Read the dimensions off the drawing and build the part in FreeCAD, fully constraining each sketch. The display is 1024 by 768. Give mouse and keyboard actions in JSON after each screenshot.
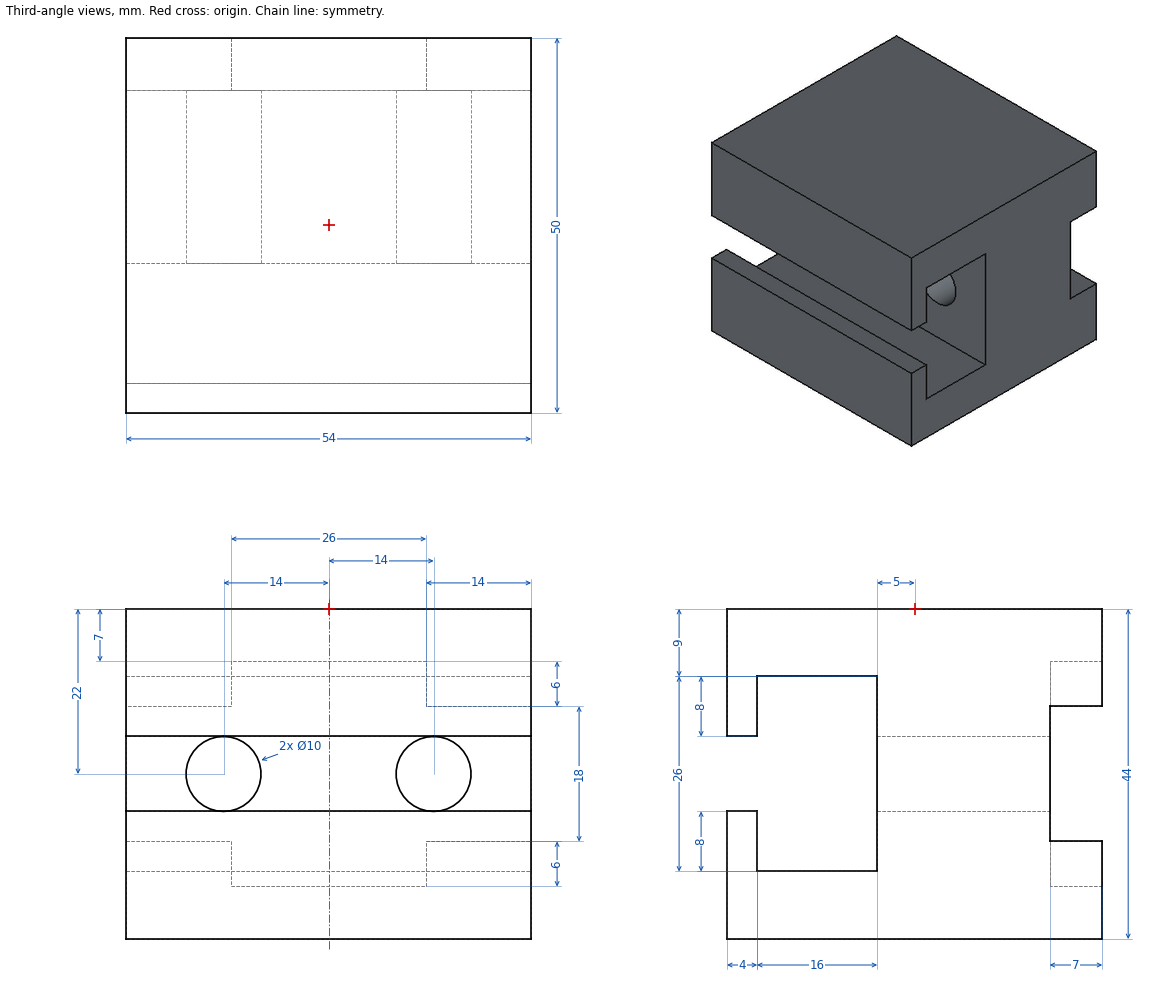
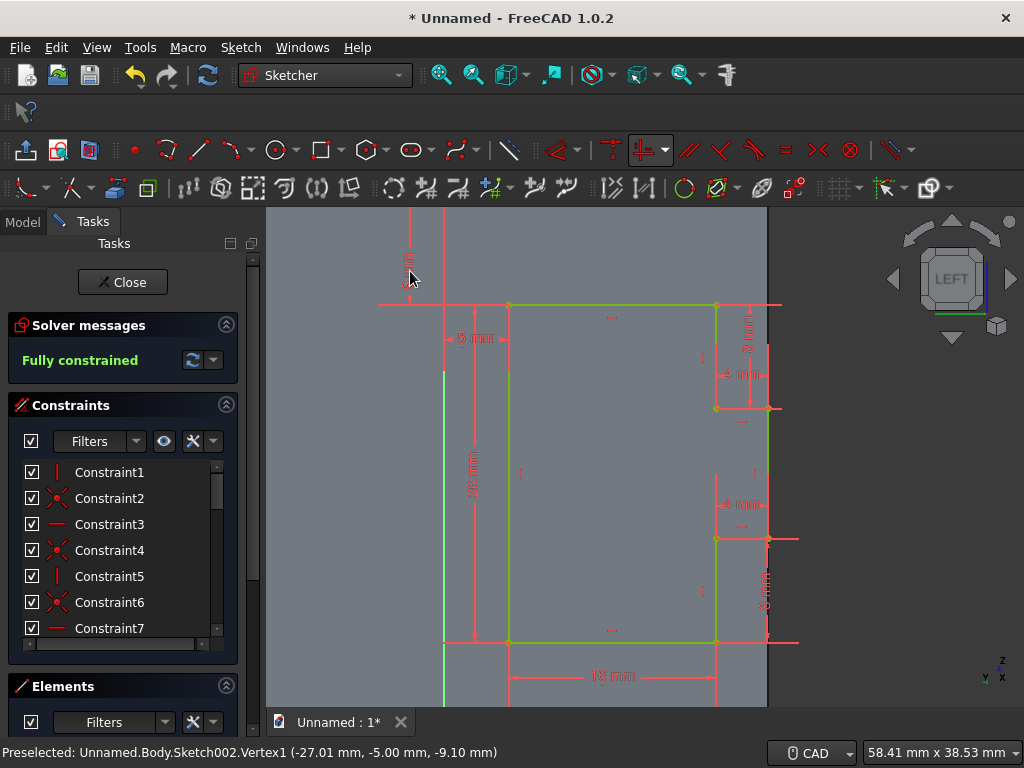
{"action": "left_click", "coordinate": [123, 282]}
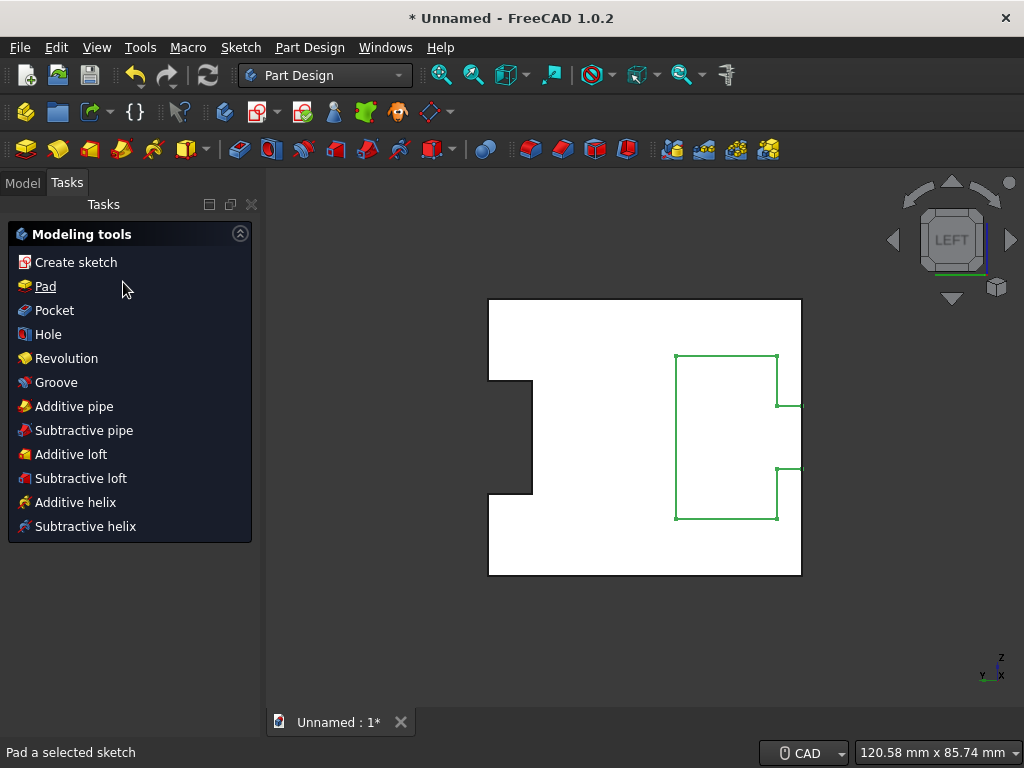
{"action": "left_click", "coordinate": [240, 150]}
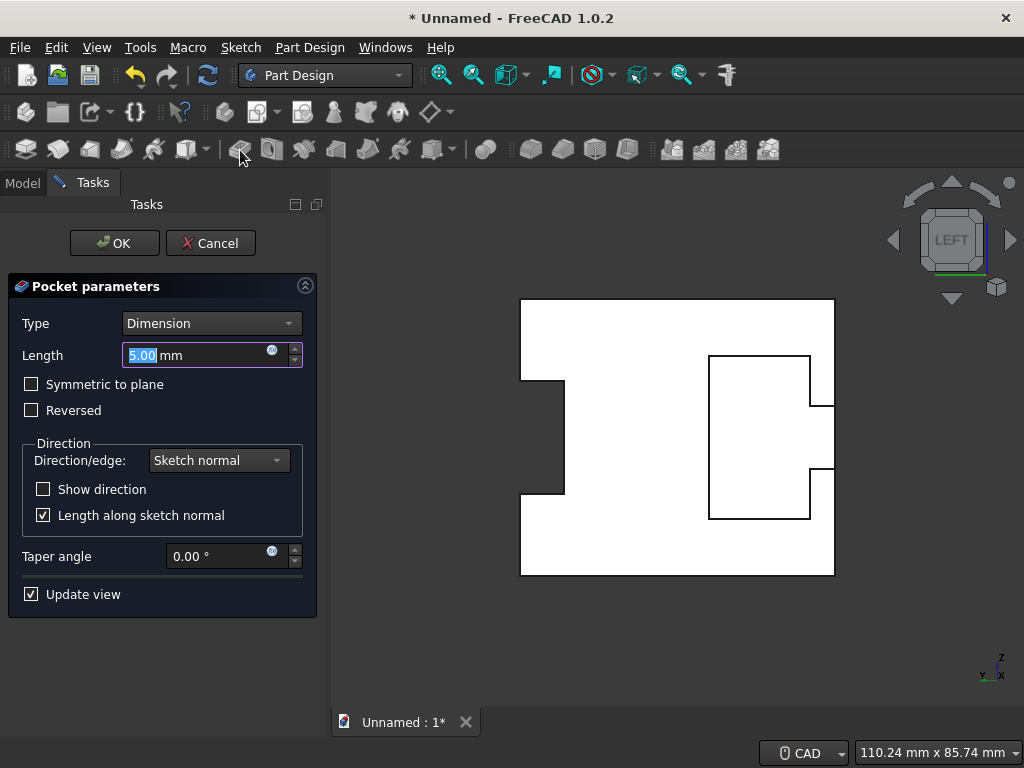
{"action": "left_click", "coordinate": [212, 324]}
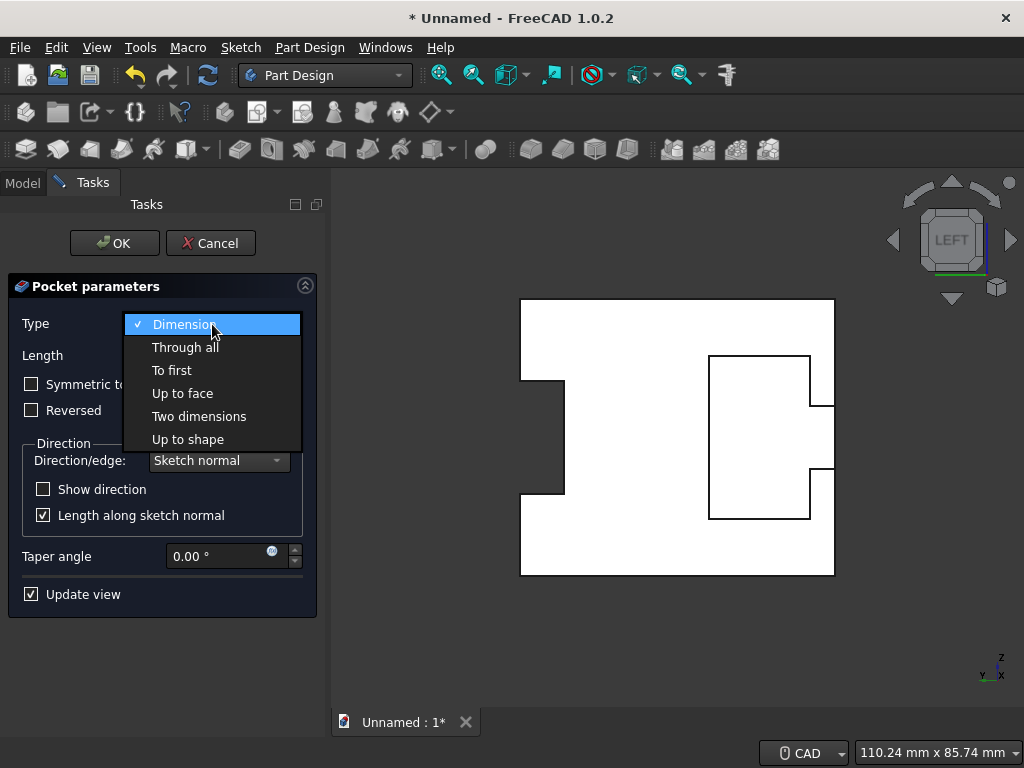
{"action": "left_click", "coordinate": [212, 348]}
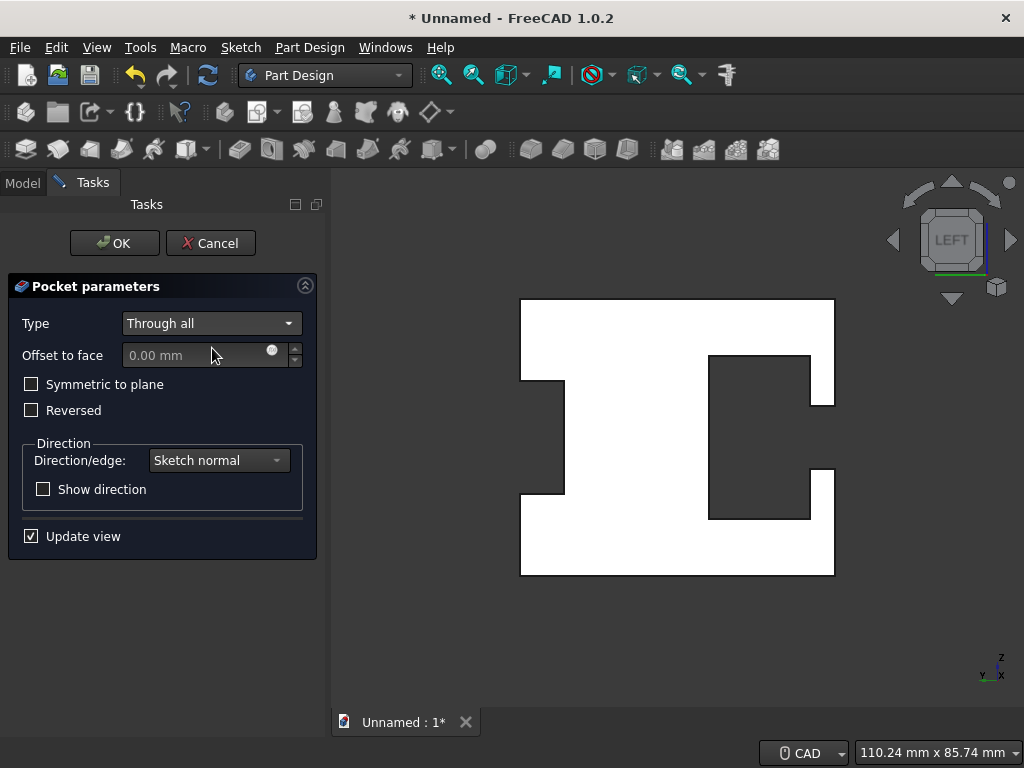
{"action": "left_click", "coordinate": [115, 243]}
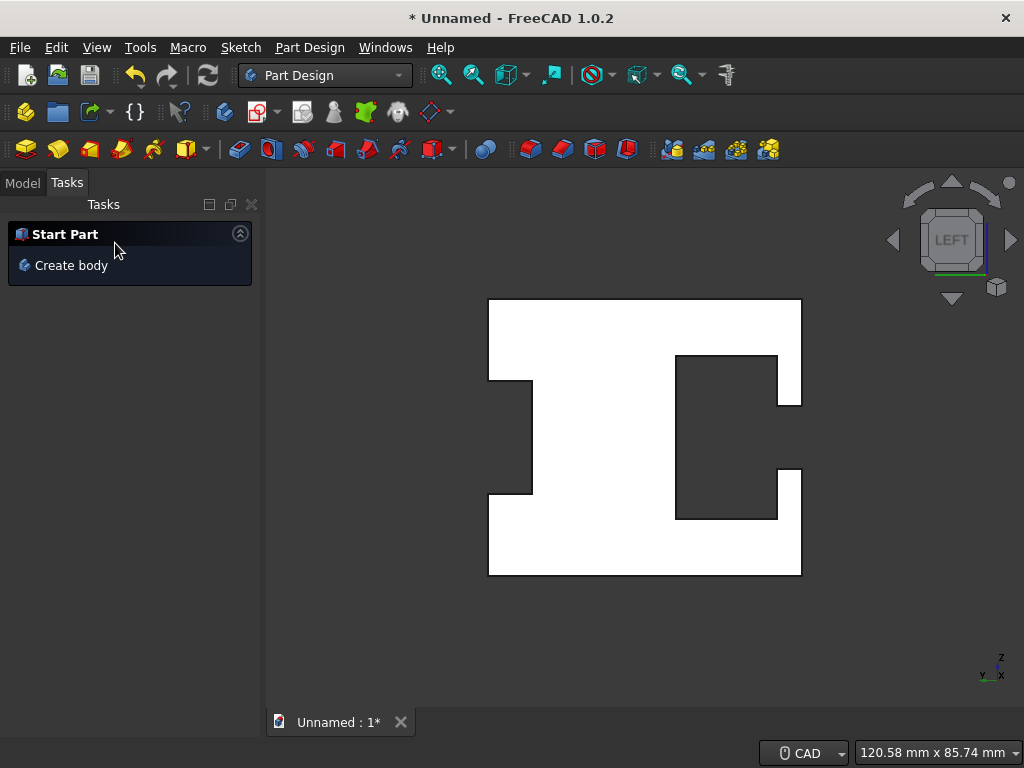
{"action": "key", "text": "4"}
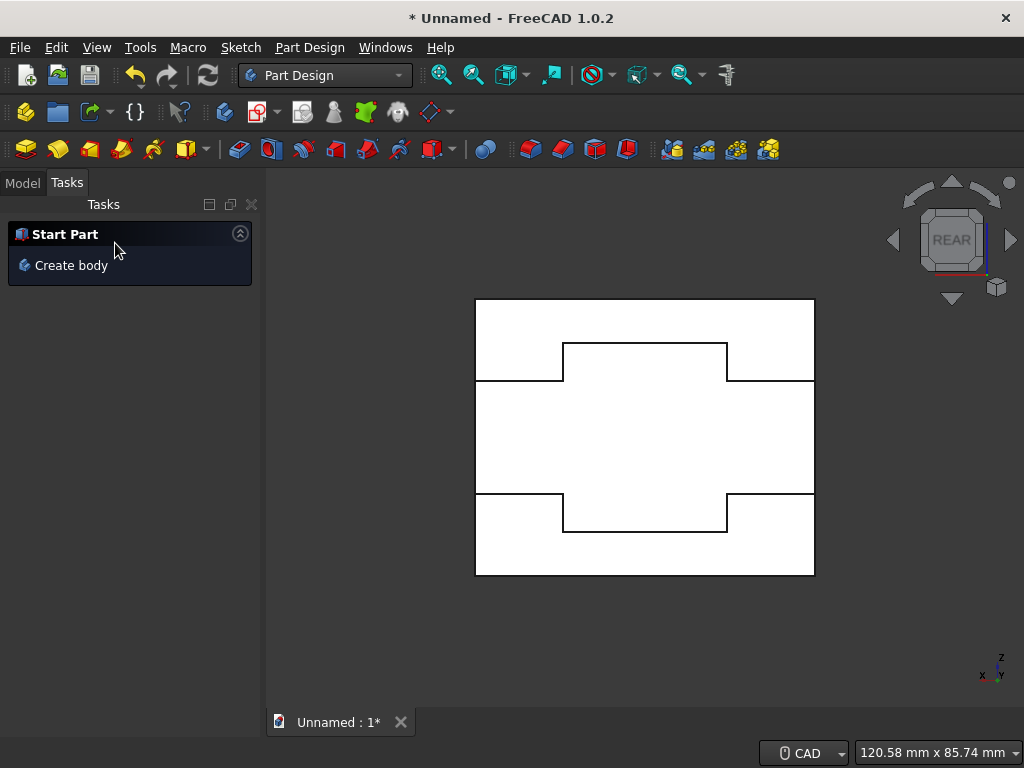
{"action": "left_click", "coordinate": [645, 437]}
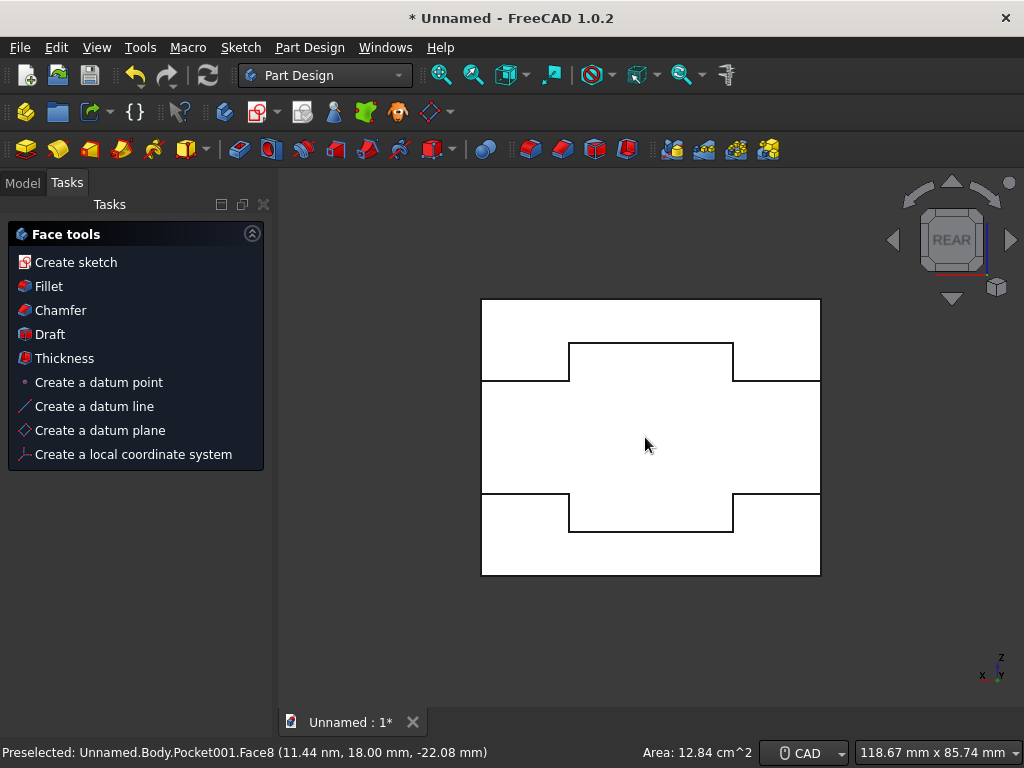
{"action": "left_click", "coordinate": [258, 112]}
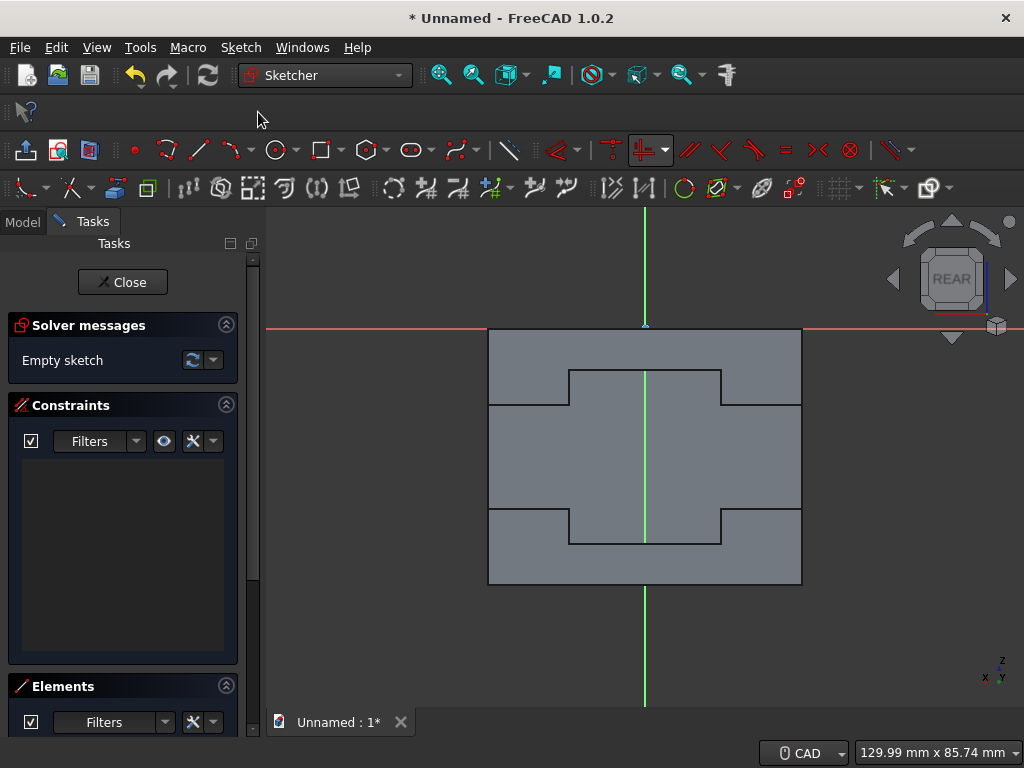
{"action": "scroll", "coordinate": [728, 347], "scroll_direction": "up", "scroll_amount": 3}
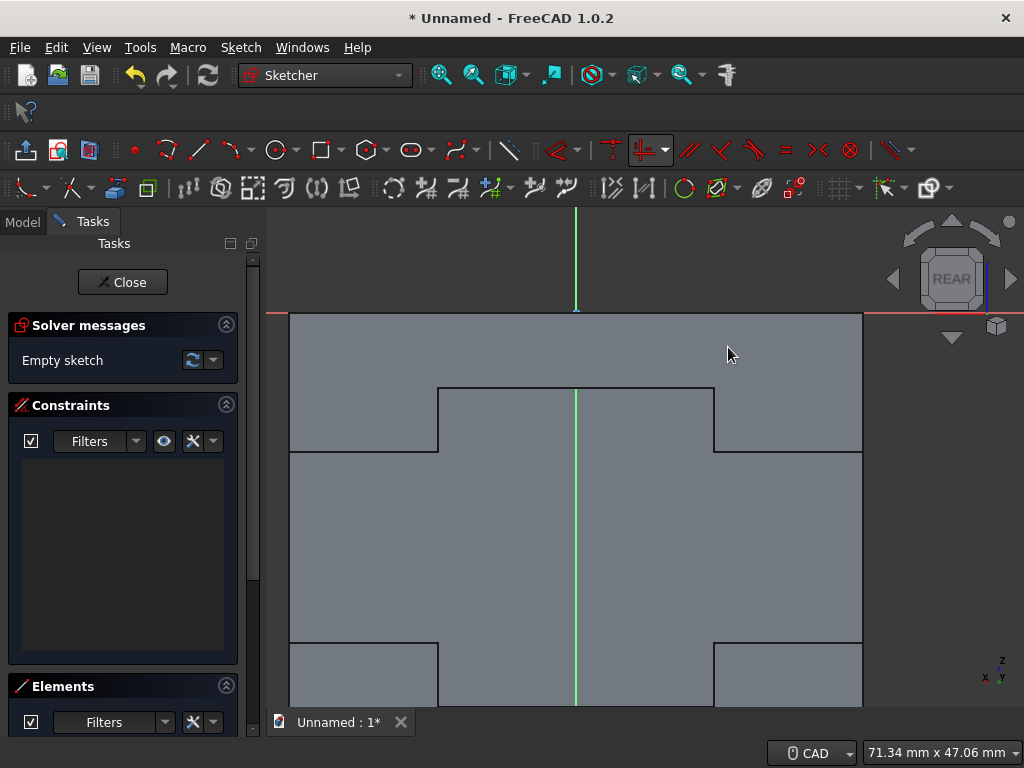
{"action": "key", "text": "g c"}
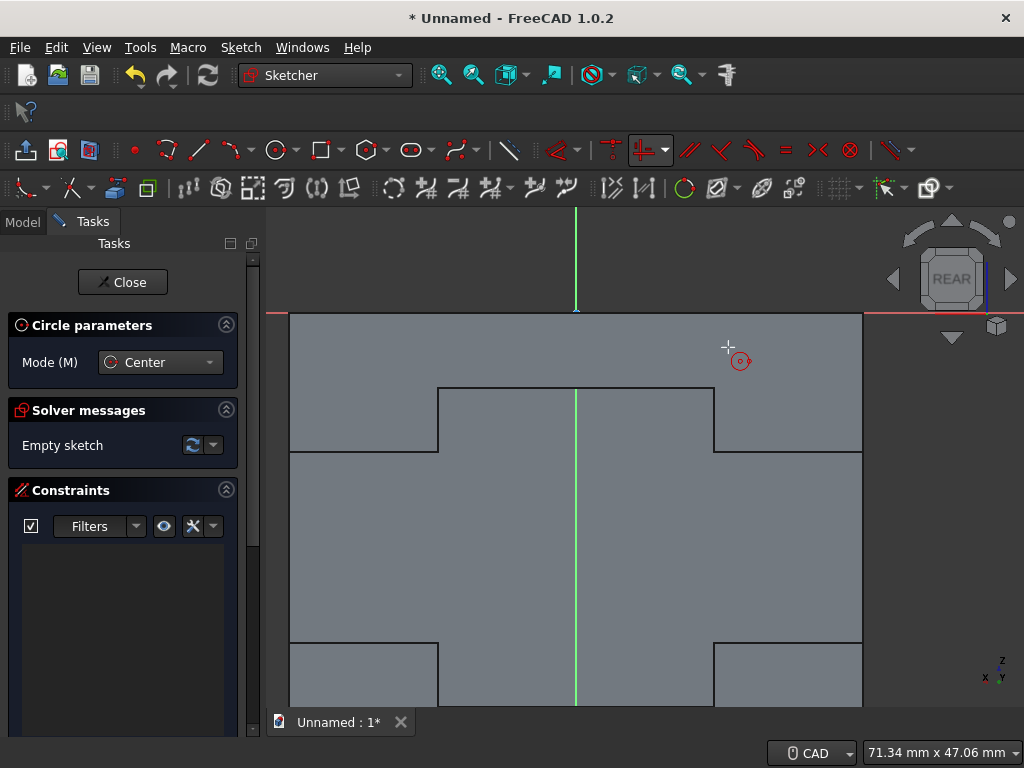
{"action": "left_click", "coordinate": [725, 547]}
{"action": "mouse_move", "coordinate": [763, 510]}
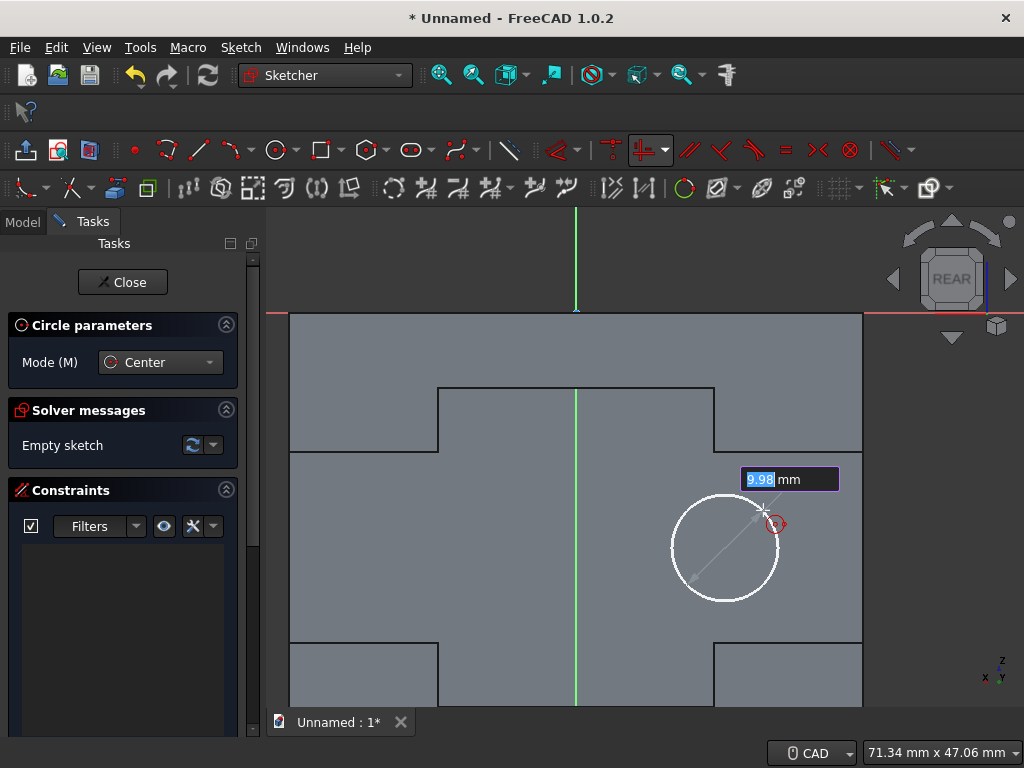
{"action": "type", "text": "10"}
{"action": "key", "text": "Return"}